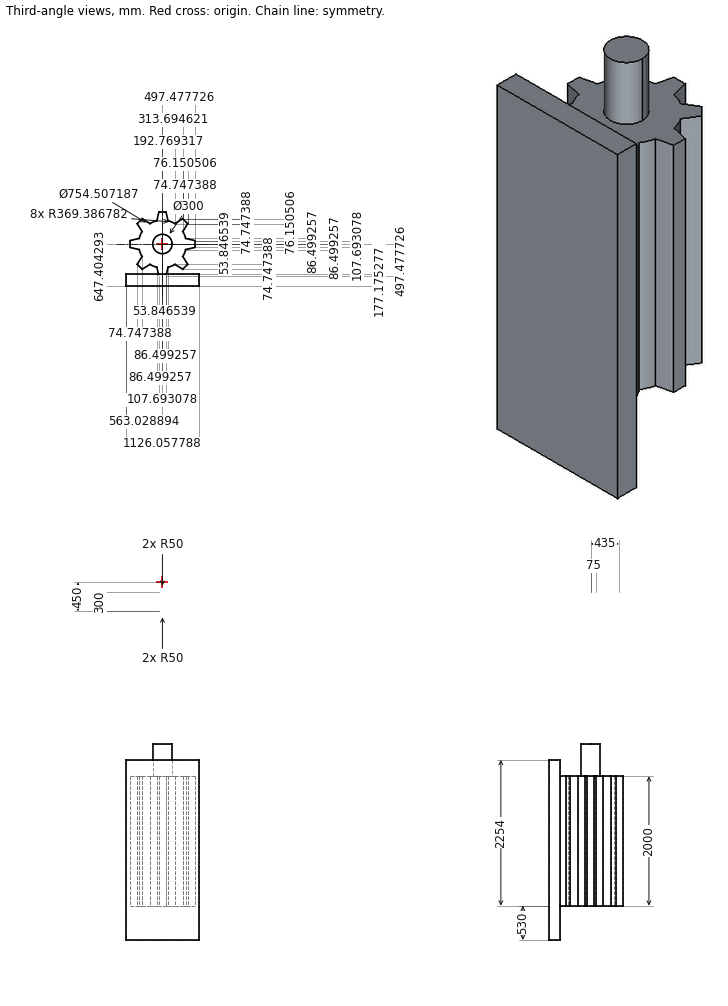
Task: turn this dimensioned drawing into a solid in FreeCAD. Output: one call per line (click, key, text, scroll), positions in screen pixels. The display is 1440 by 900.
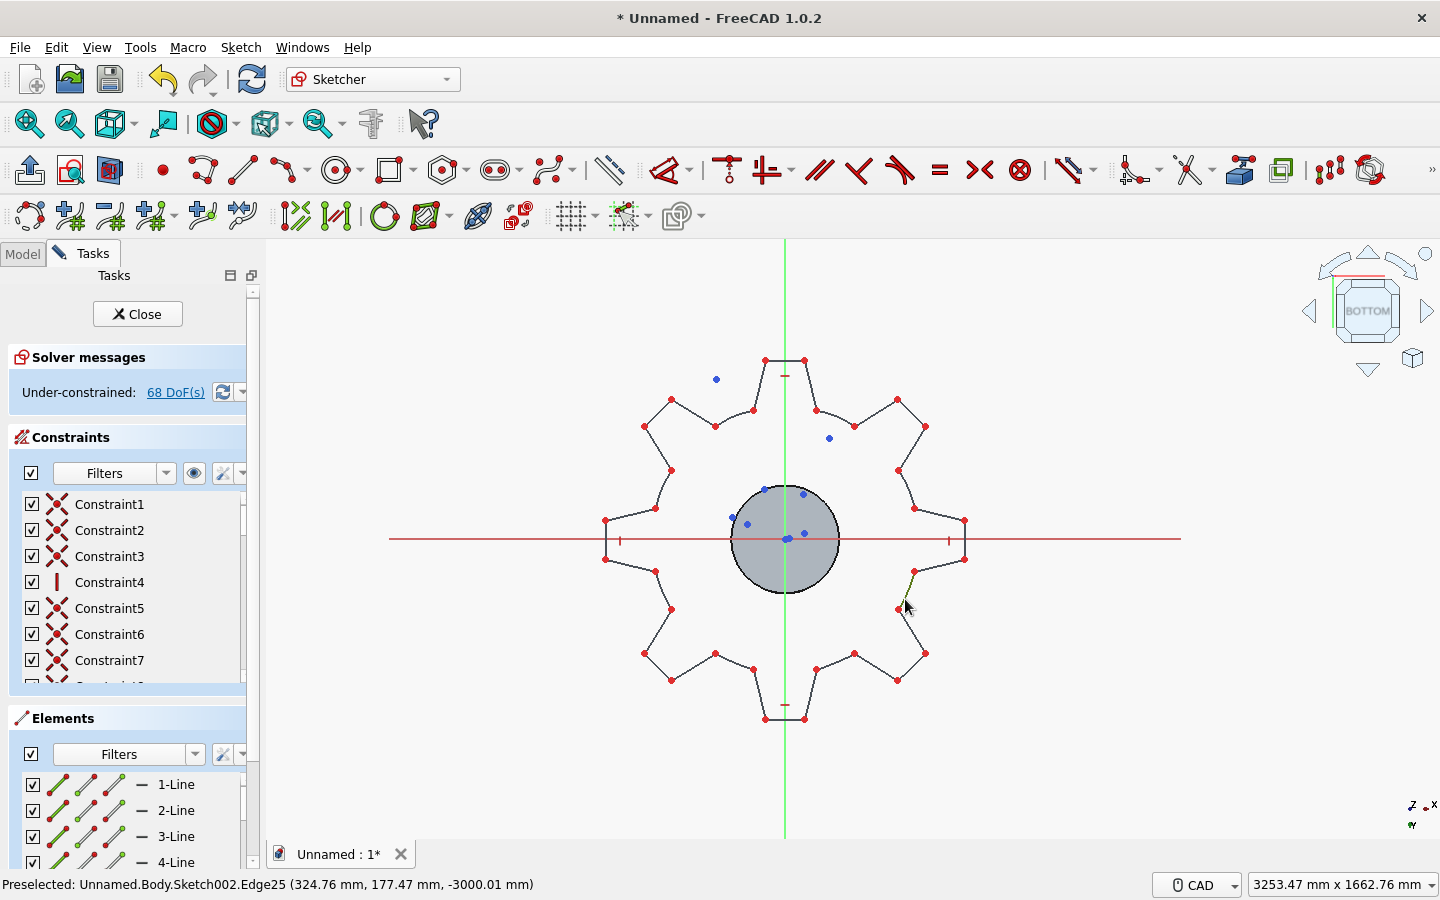
click(912, 497)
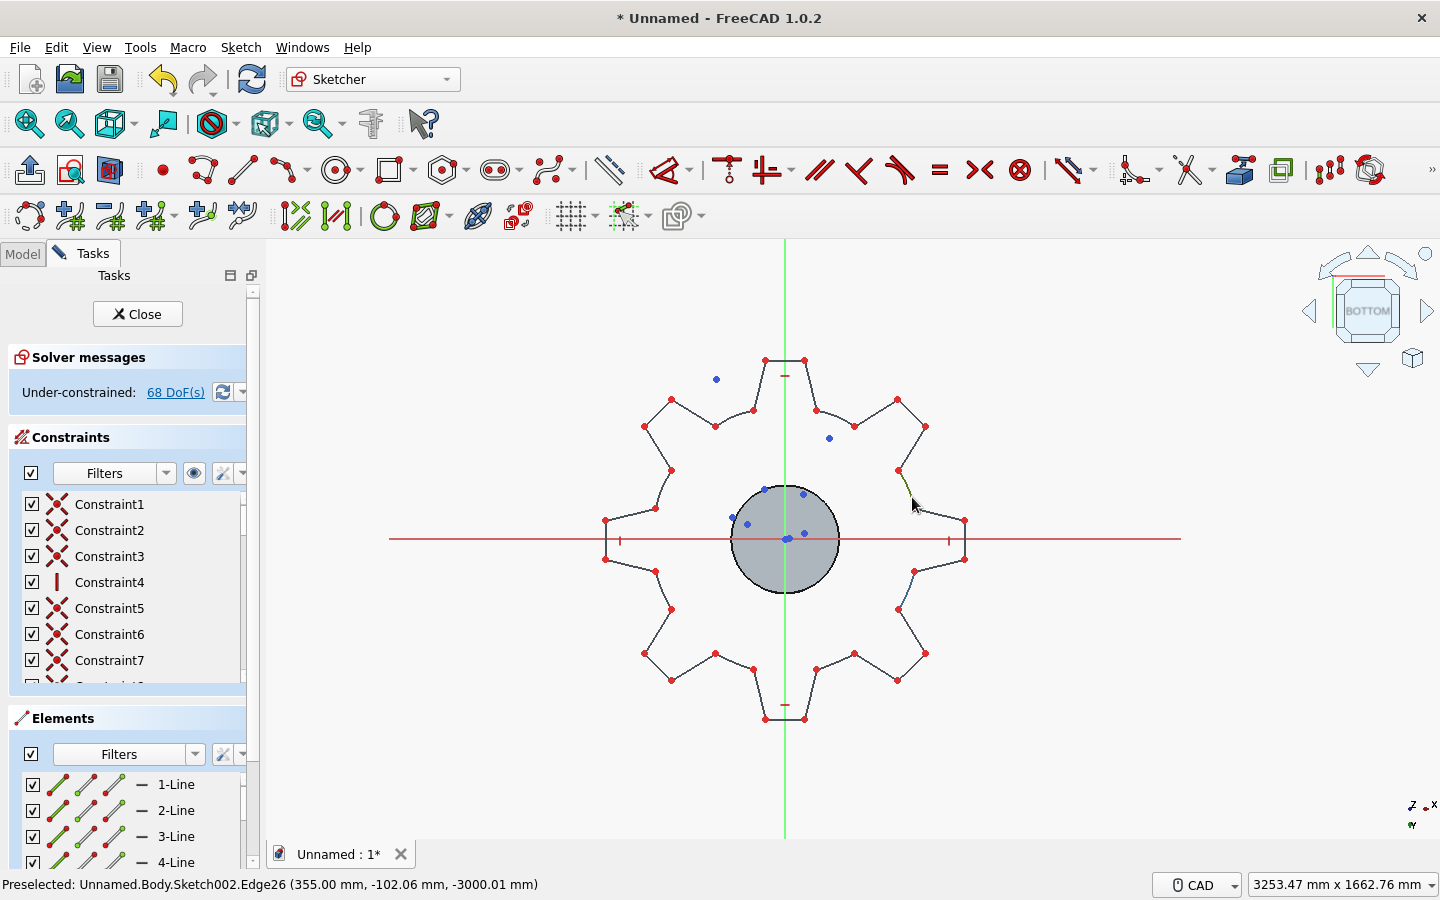
click(728, 170)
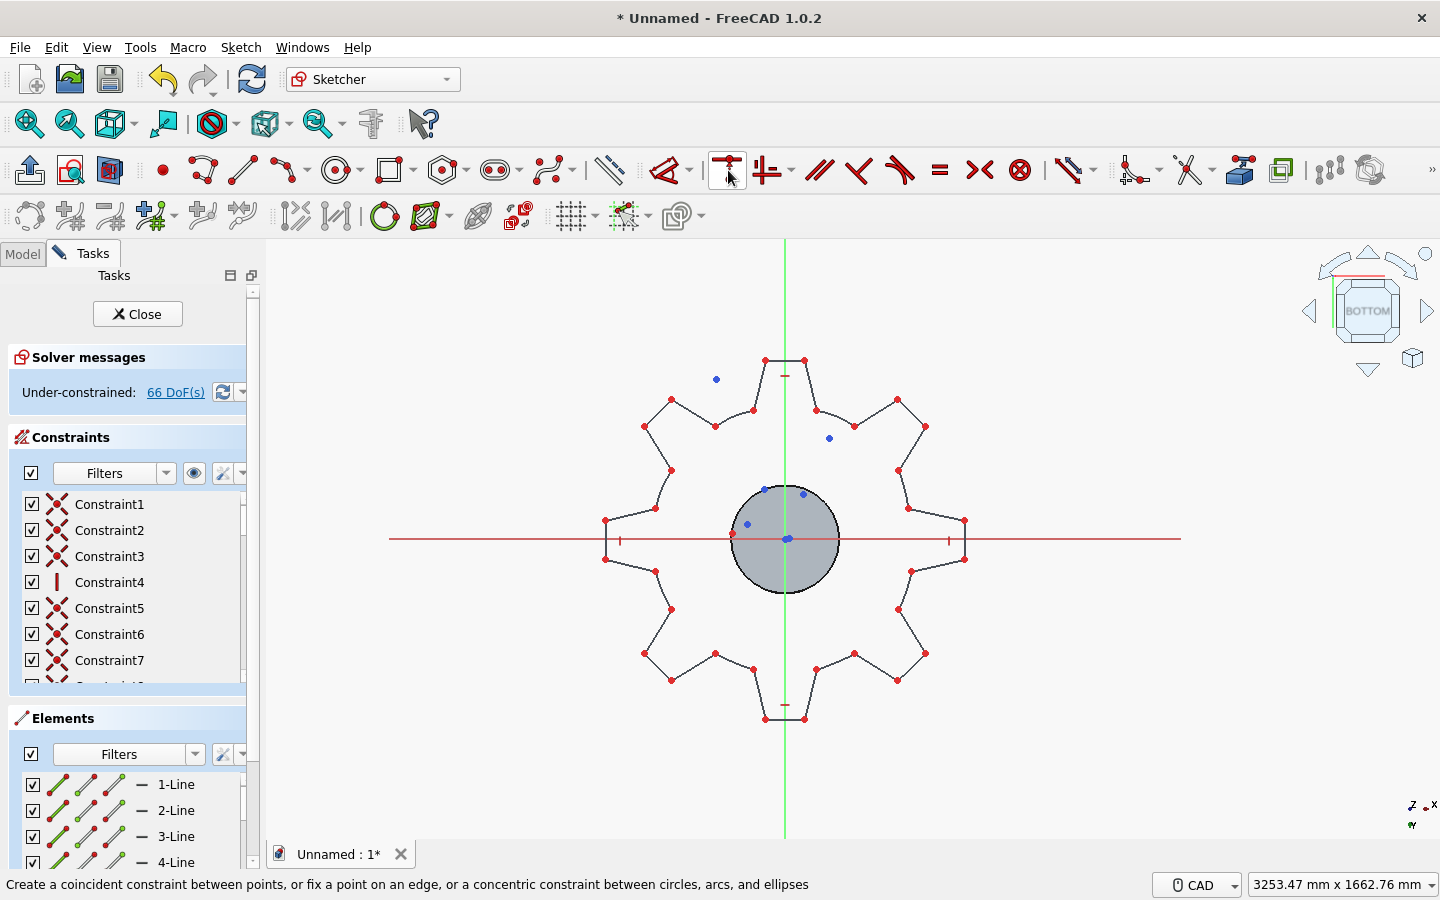
click(904, 599)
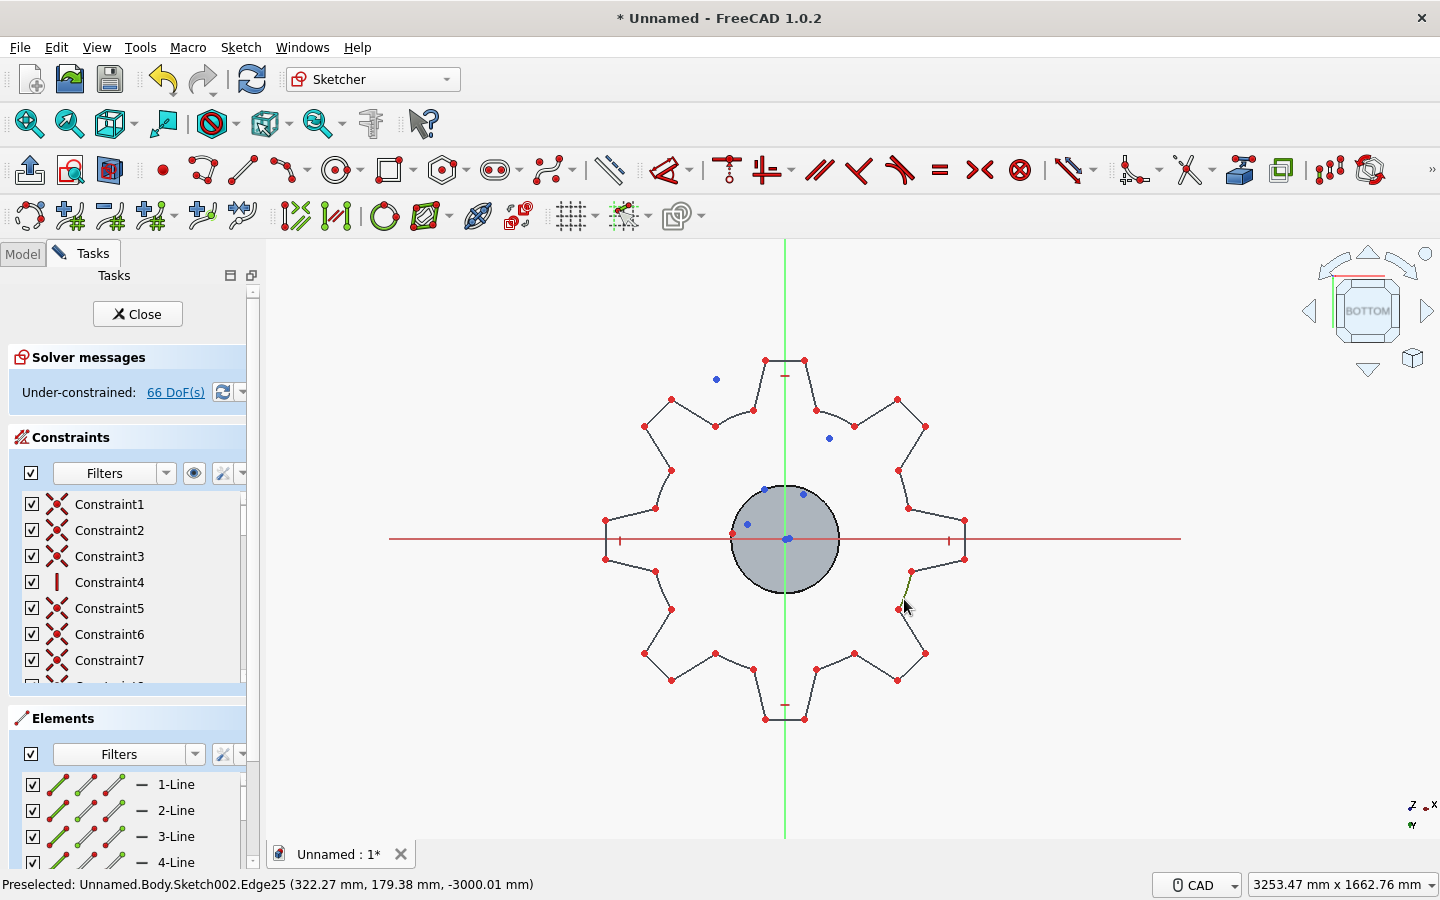
click(844, 420)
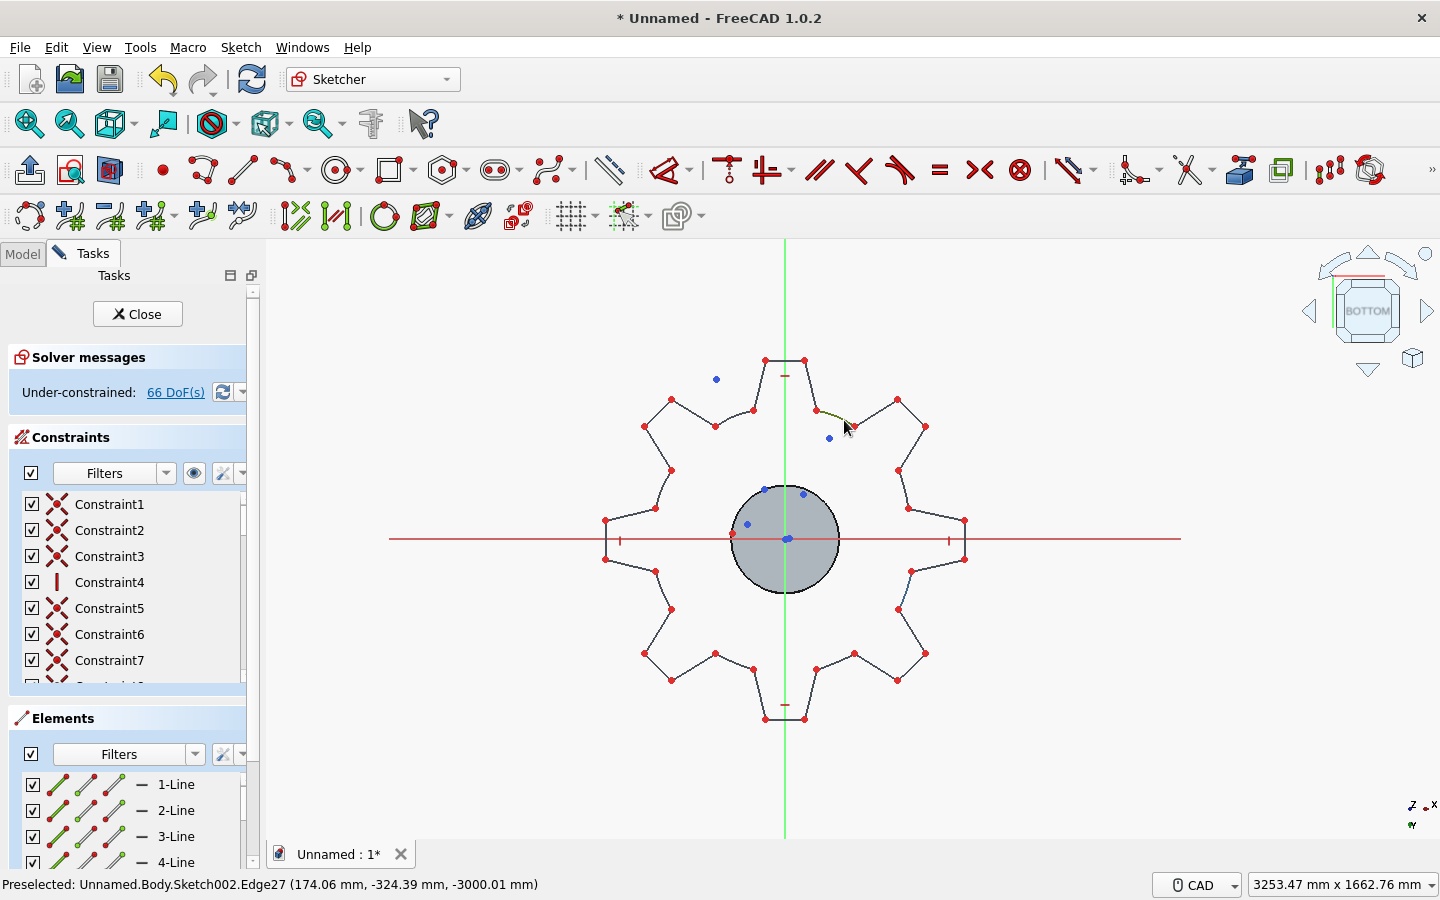
click(728, 170)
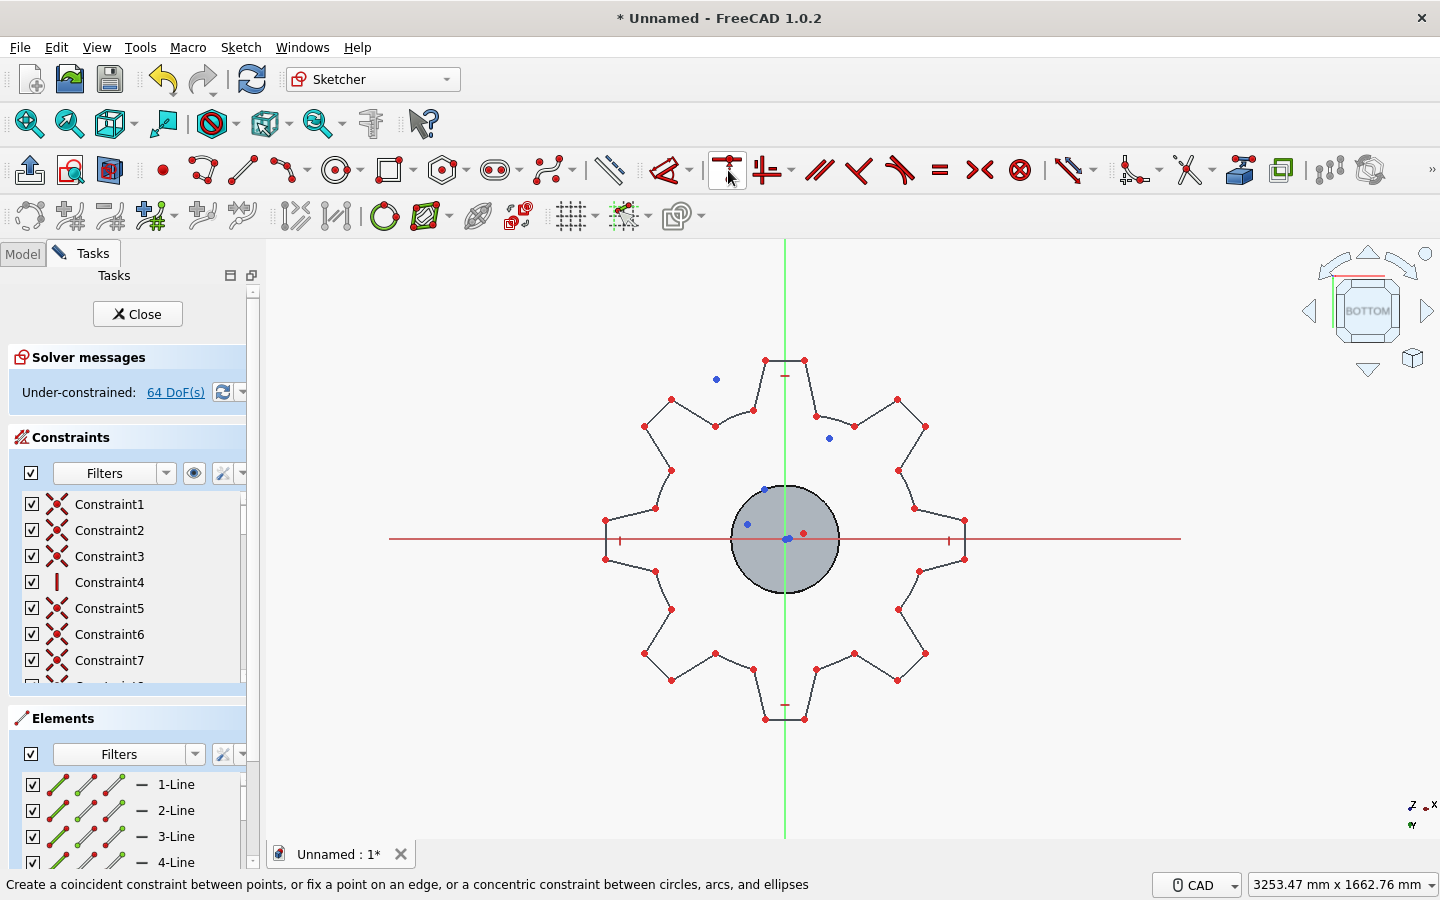
click(907, 599)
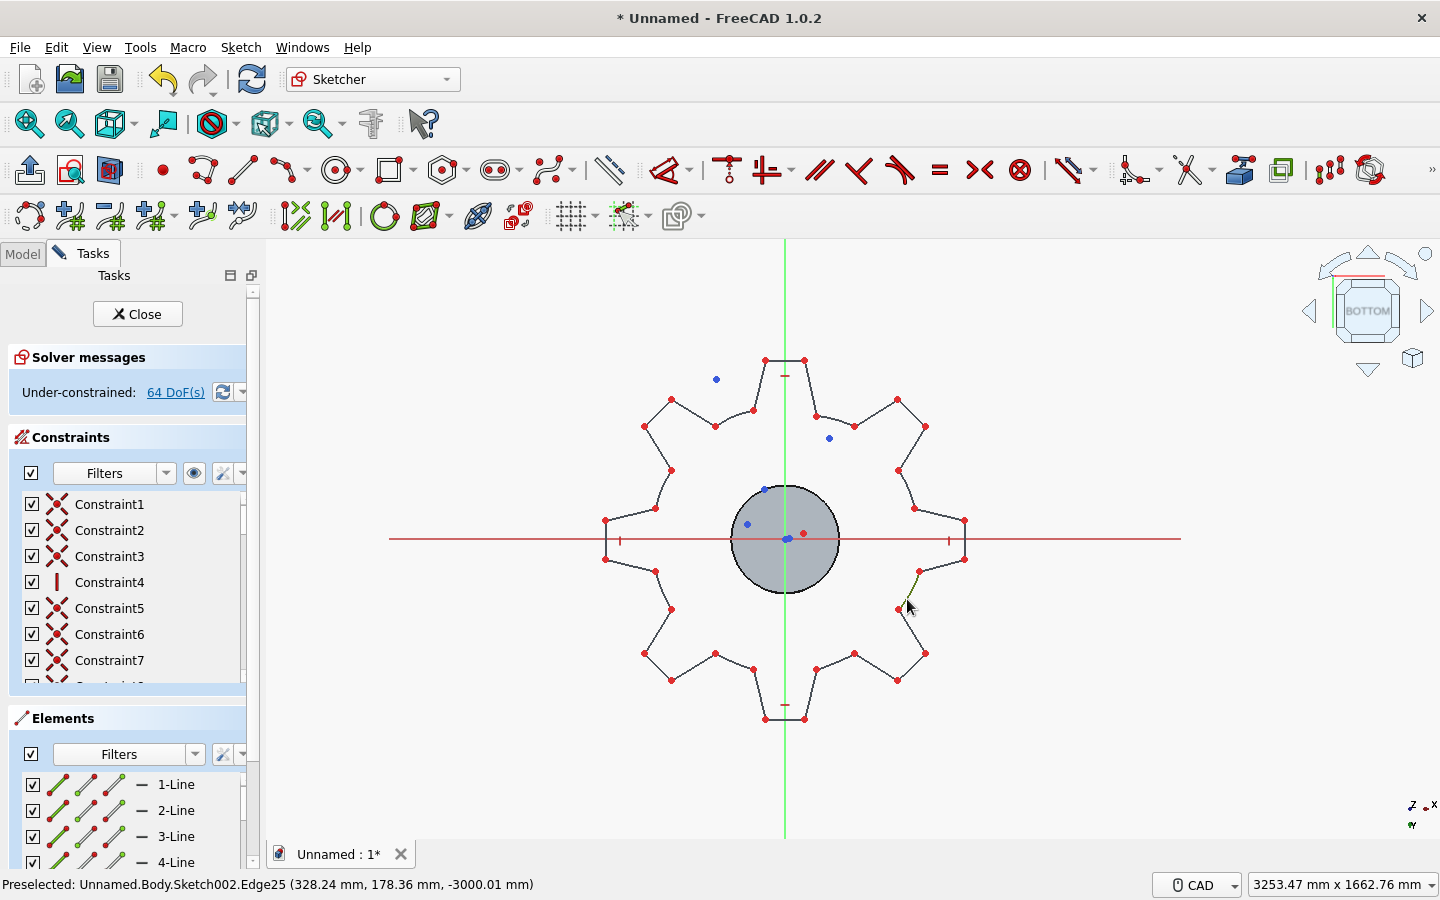
click(742, 414)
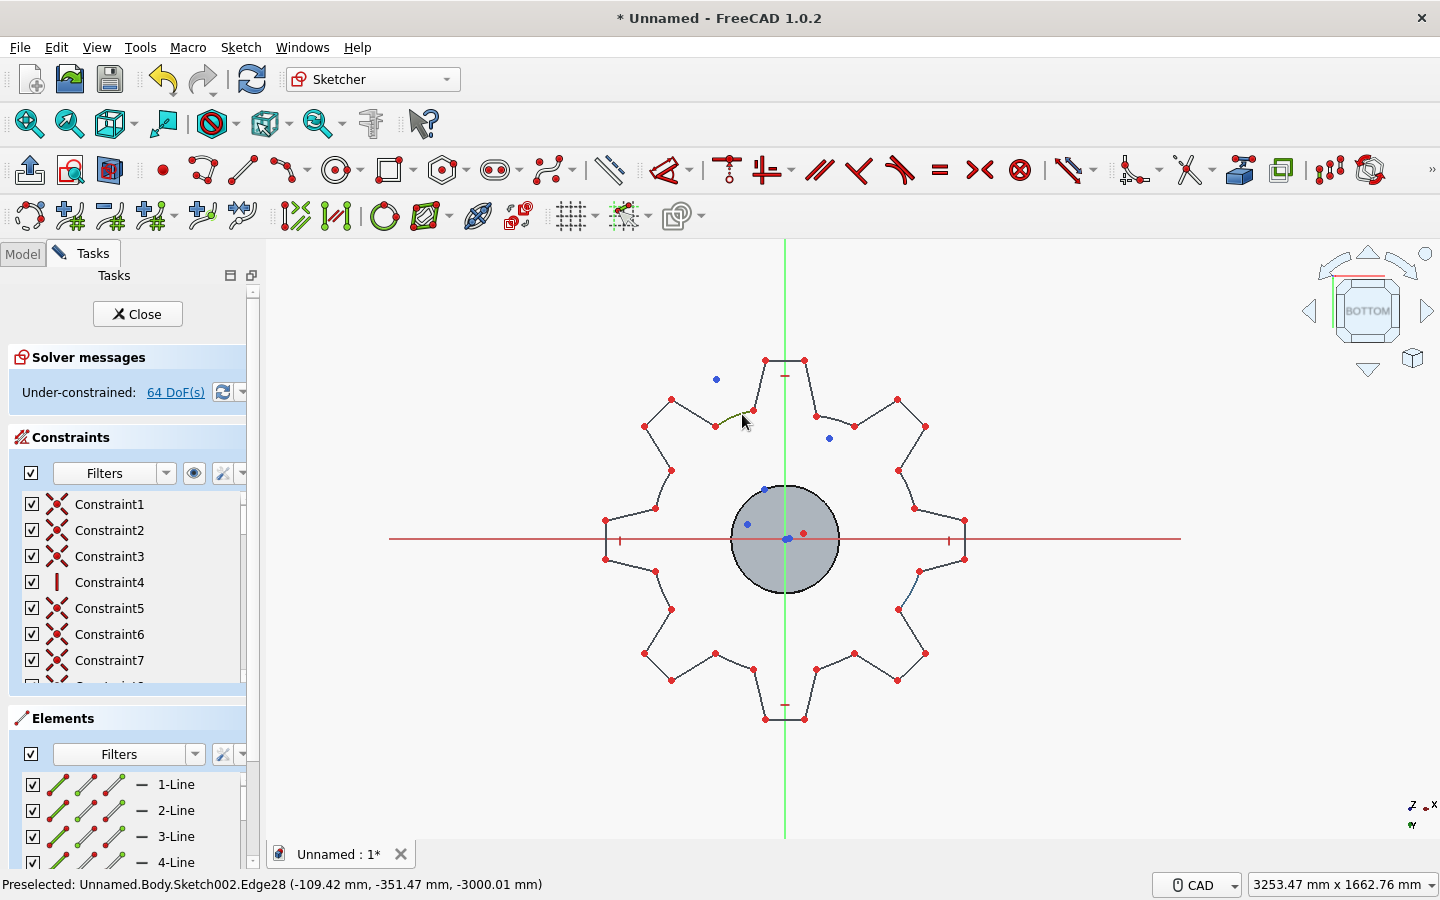
click(728, 170)